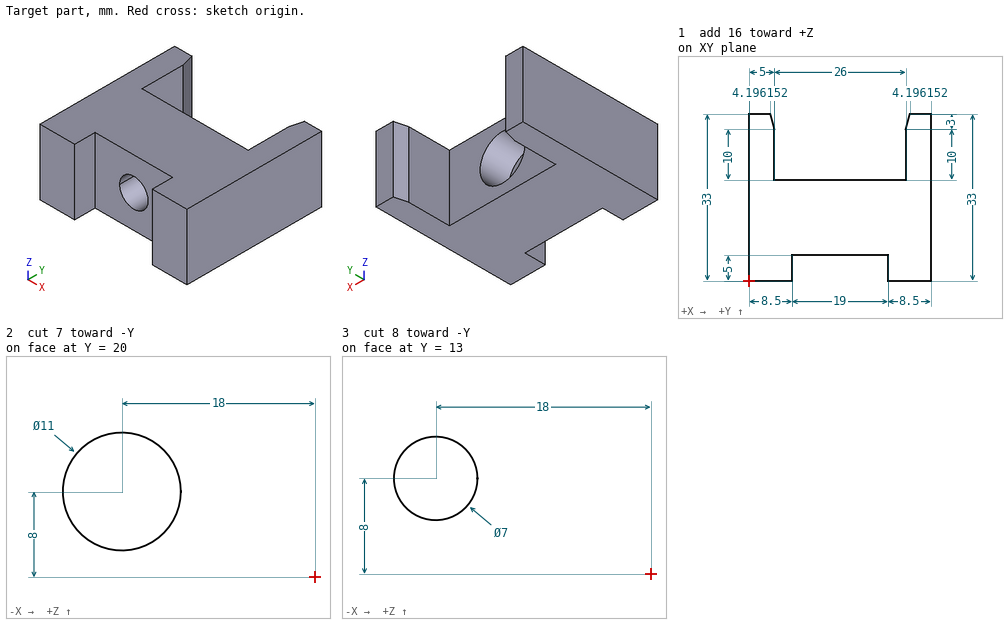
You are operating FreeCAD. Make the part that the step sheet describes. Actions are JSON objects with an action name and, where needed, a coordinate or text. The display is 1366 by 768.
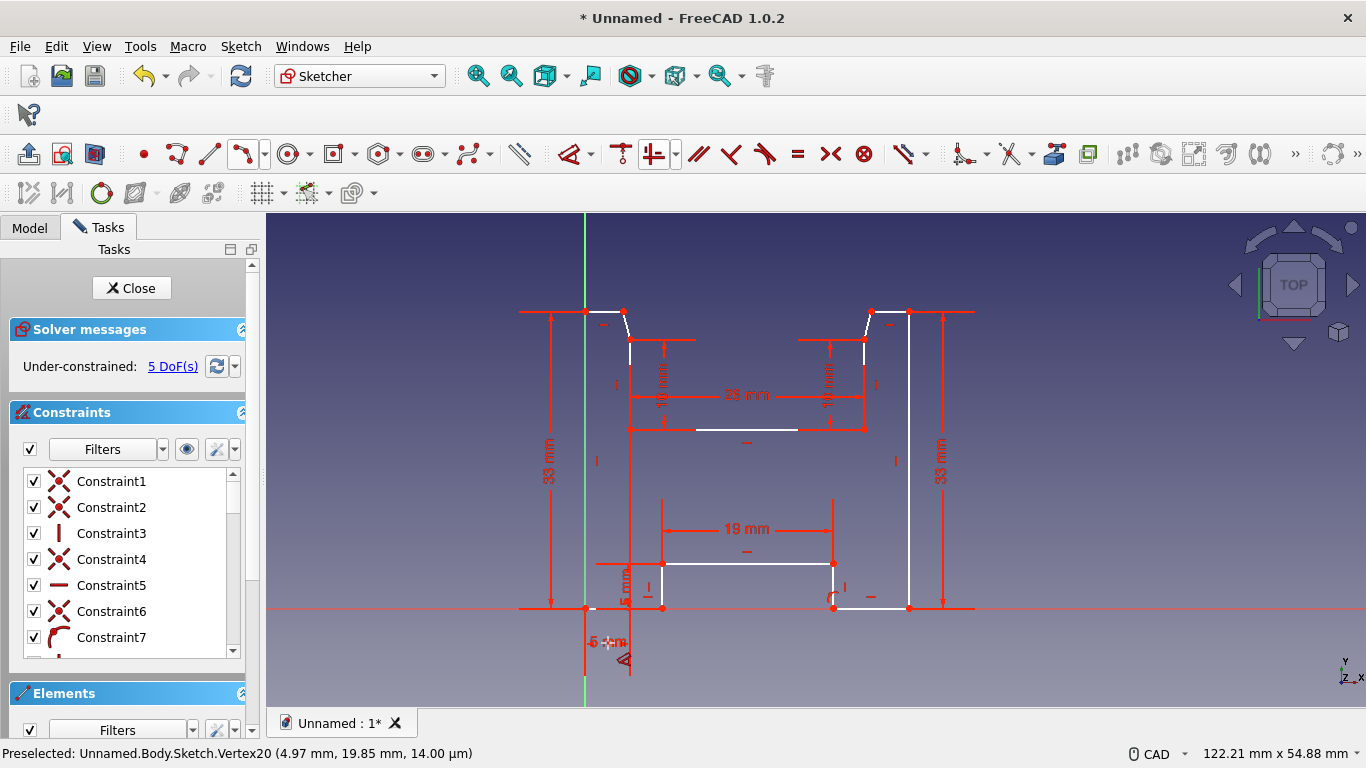
{"action": "scroll", "coordinate": [868, 323], "scroll_direction": "up", "scroll_amount": 2}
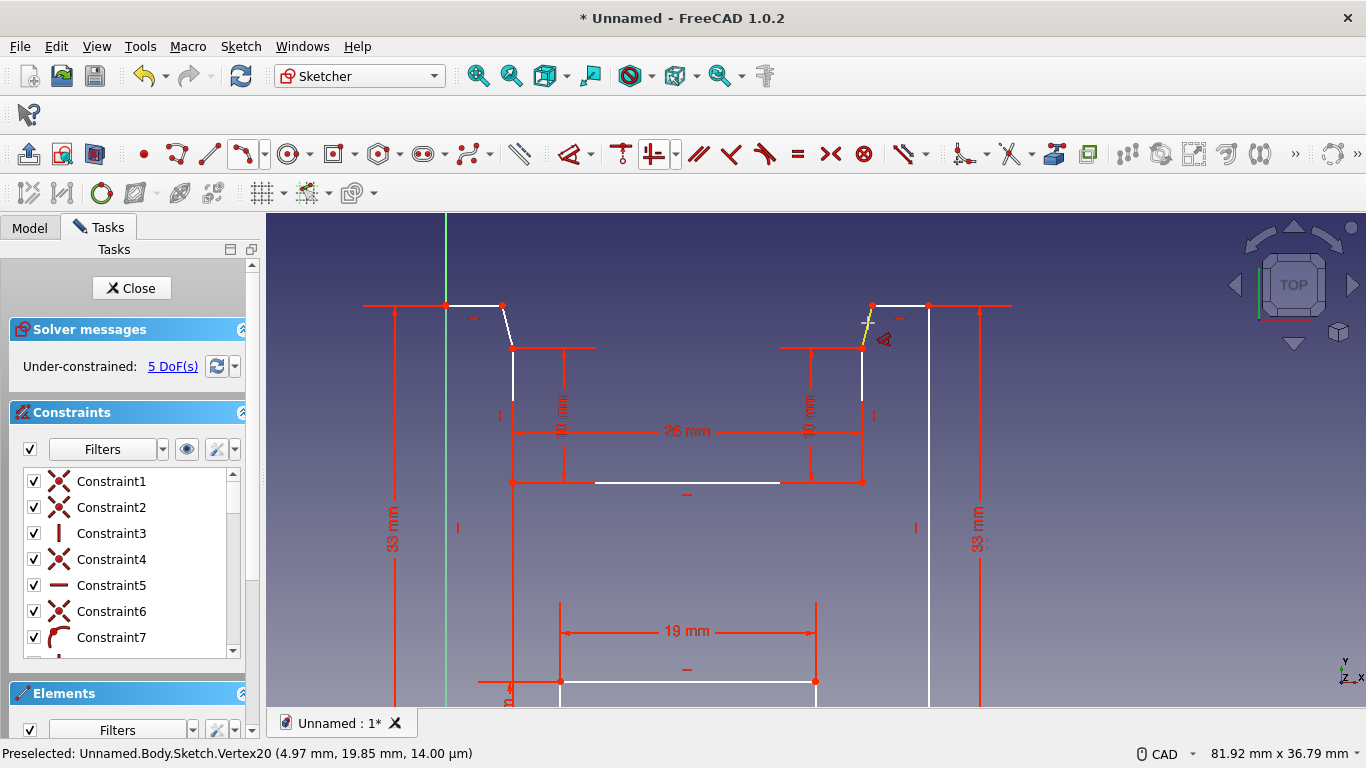
{"action": "left_click", "coordinate": [868, 323]}
{"action": "left_click", "coordinate": [906, 327]}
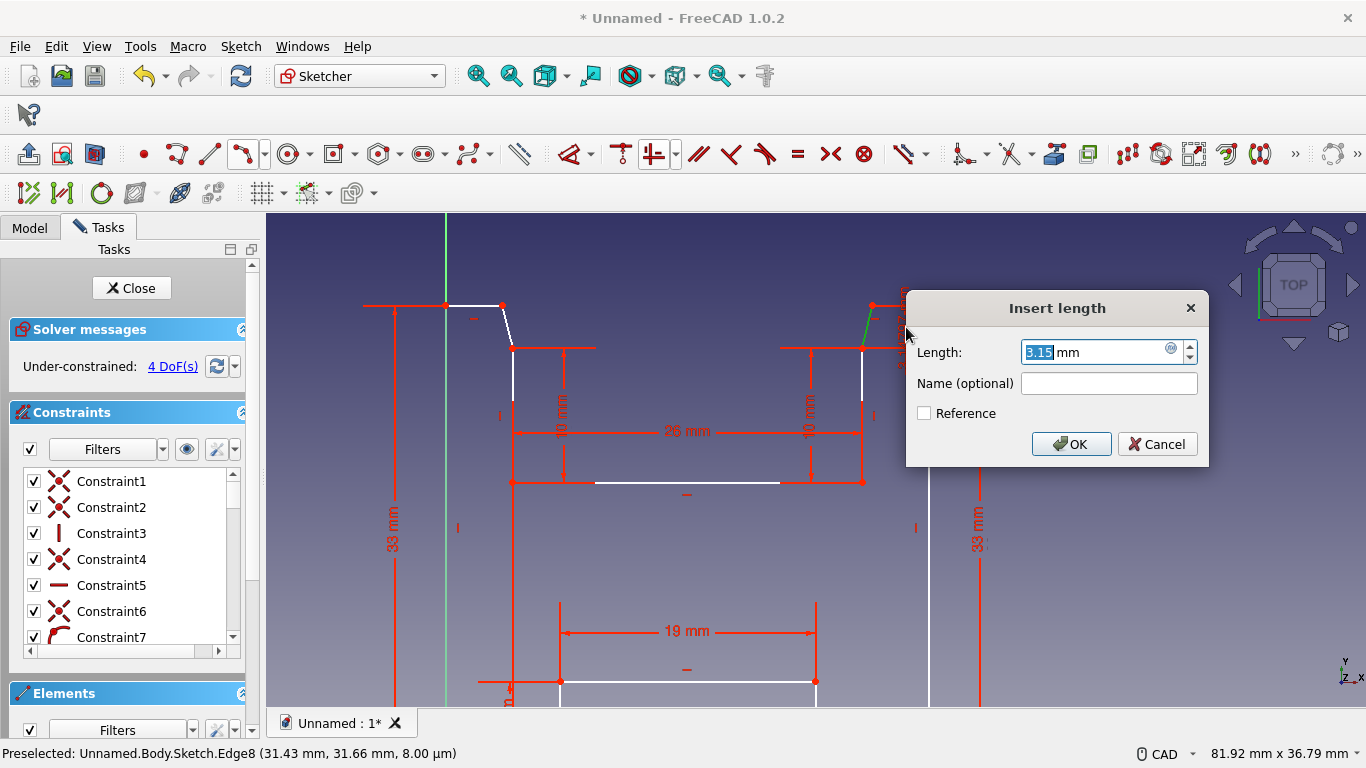
{"action": "type", "text": "3"}
{"action": "key", "text": "Return"}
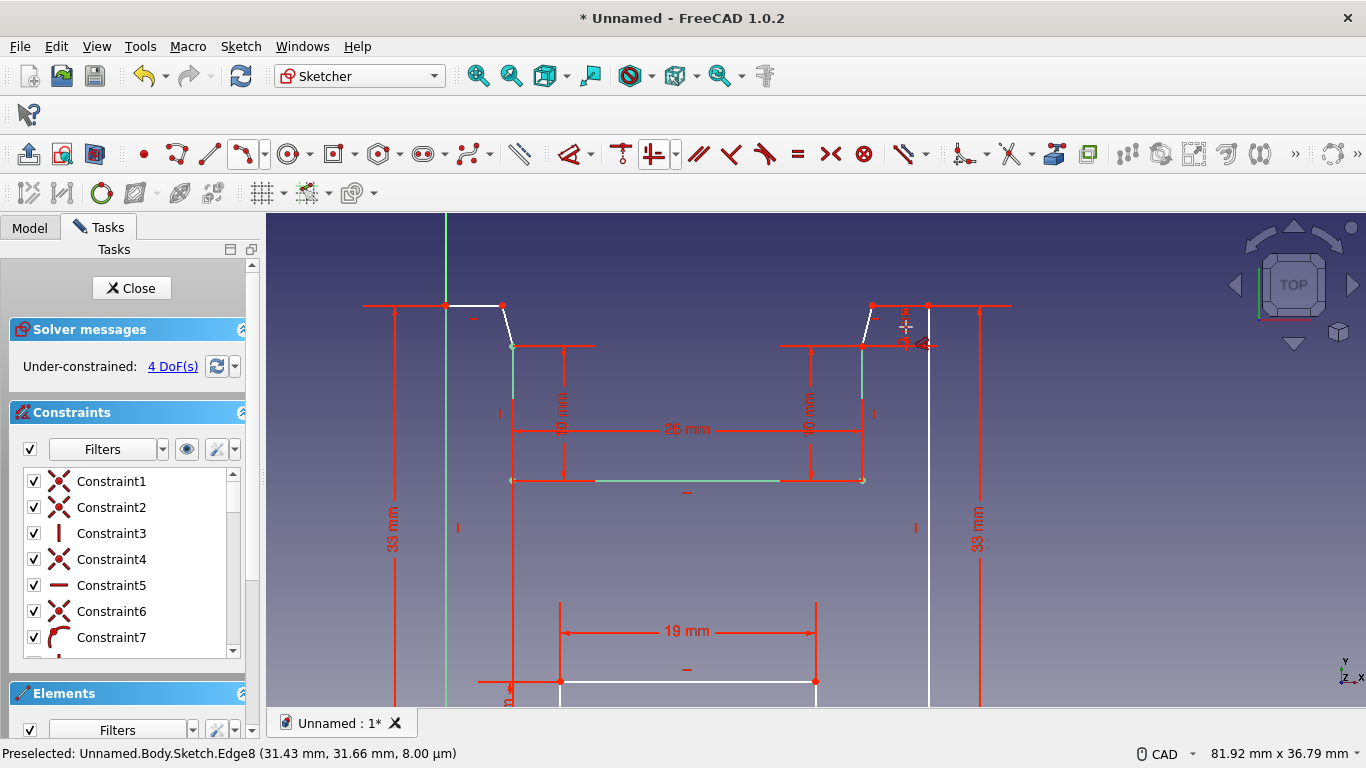
{"action": "scroll", "coordinate": [869, 323], "scroll_direction": "down", "scroll_amount": 2}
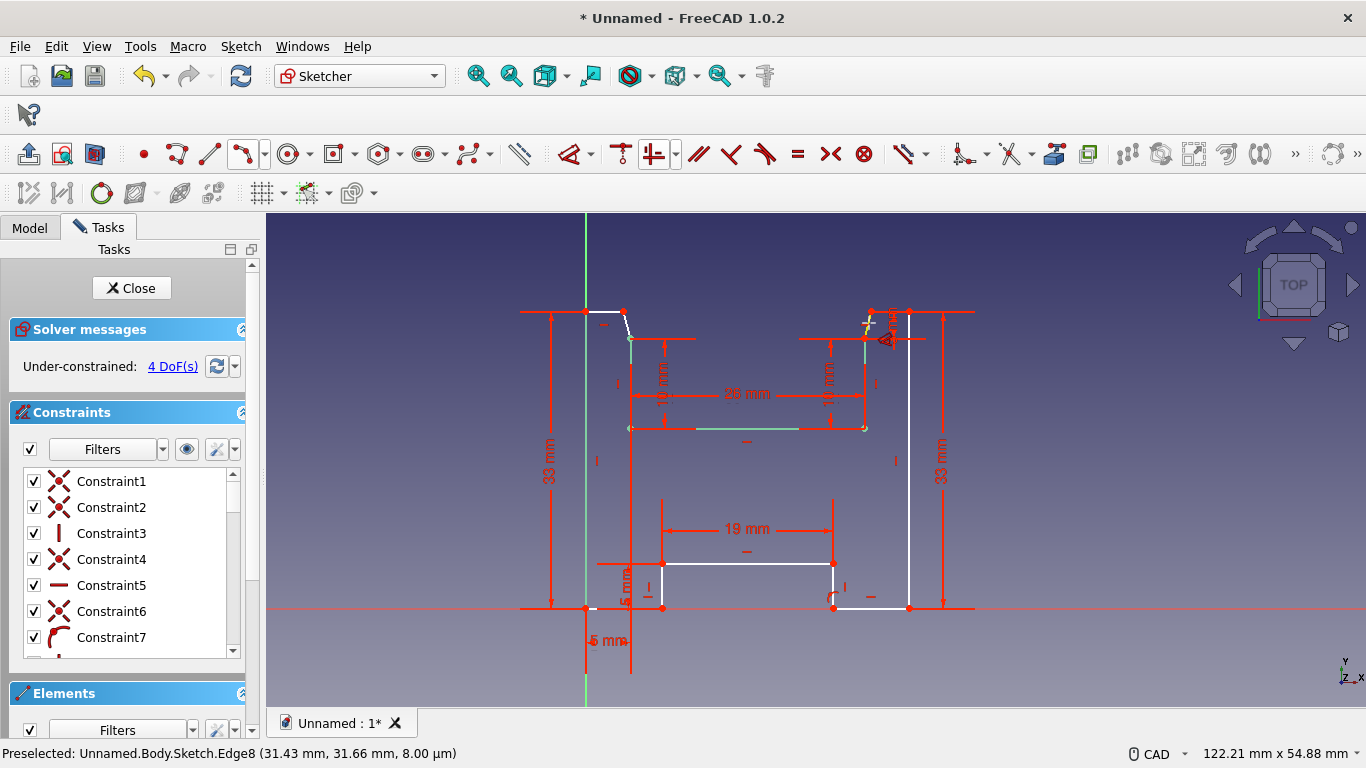
{"action": "left_click", "coordinate": [609, 609]}
{"action": "left_click", "coordinate": [624, 667]}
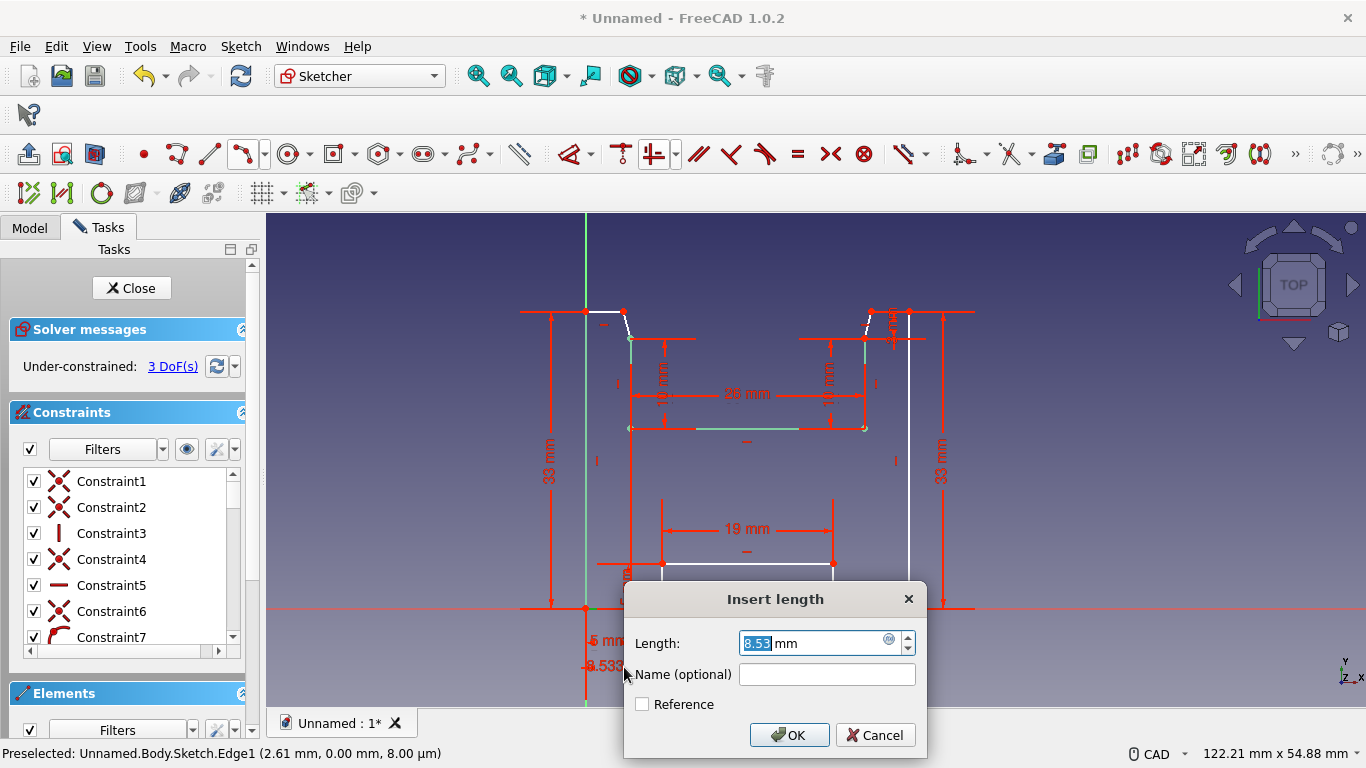
{"action": "type", "text": "8.5"}
{"action": "key", "text": "Return"}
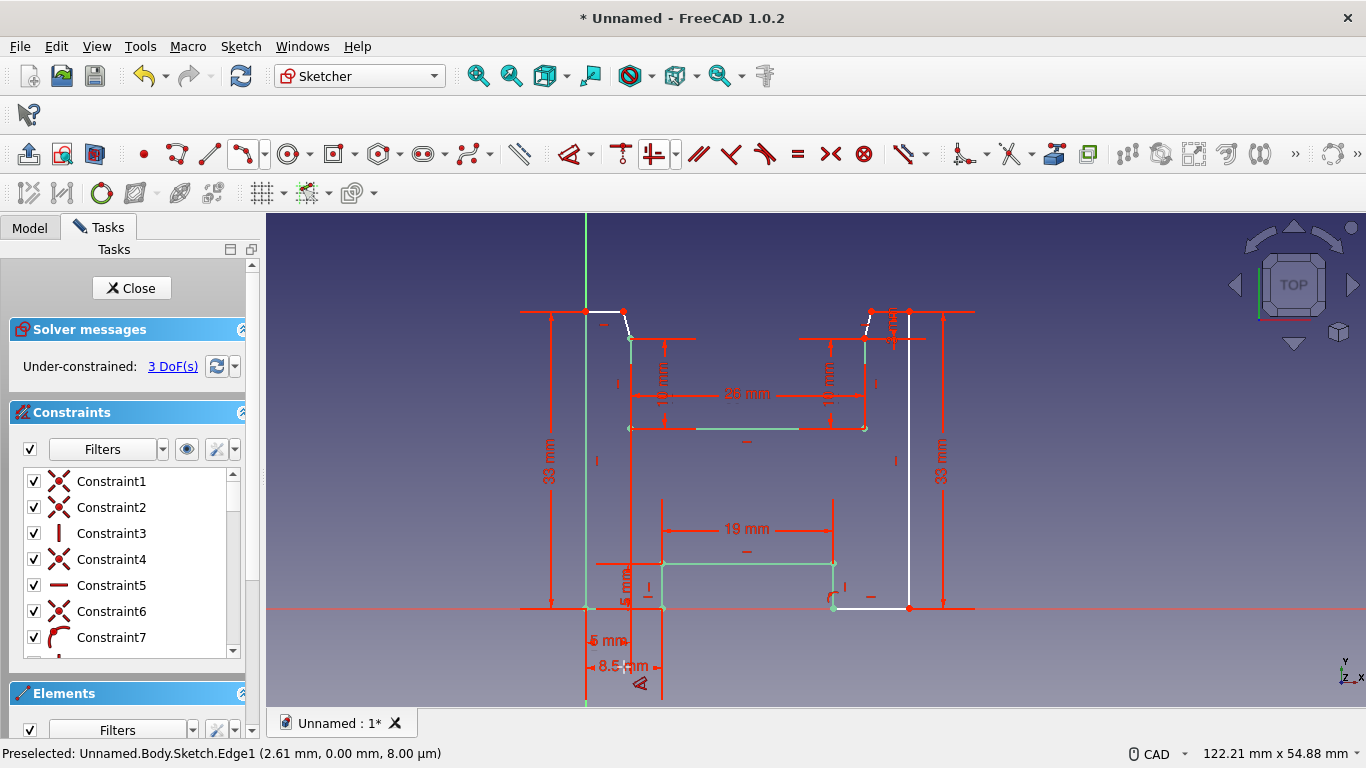
{"action": "left_click", "coordinate": [856, 609]}
{"action": "left_click", "coordinate": [871, 643]}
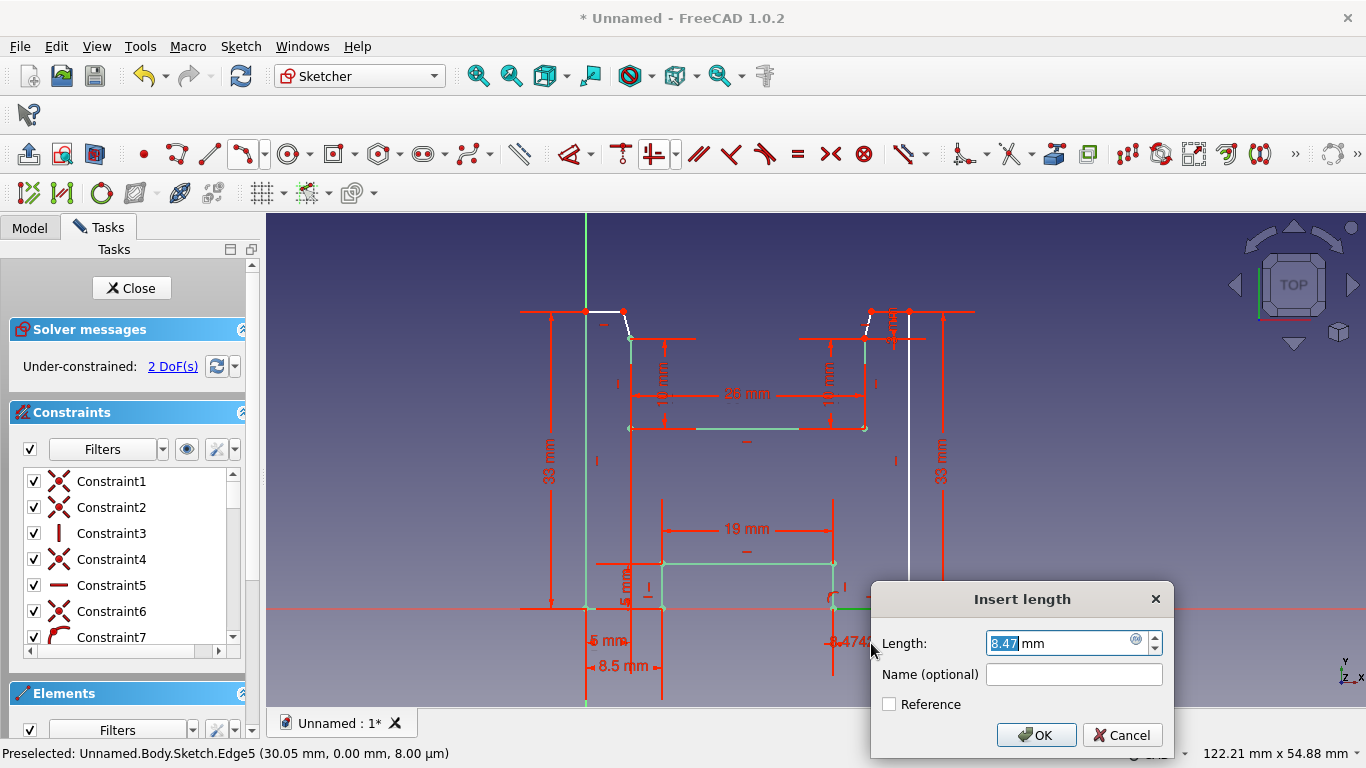
{"action": "type", "text": "8.5"}
{"action": "key", "text": "Return"}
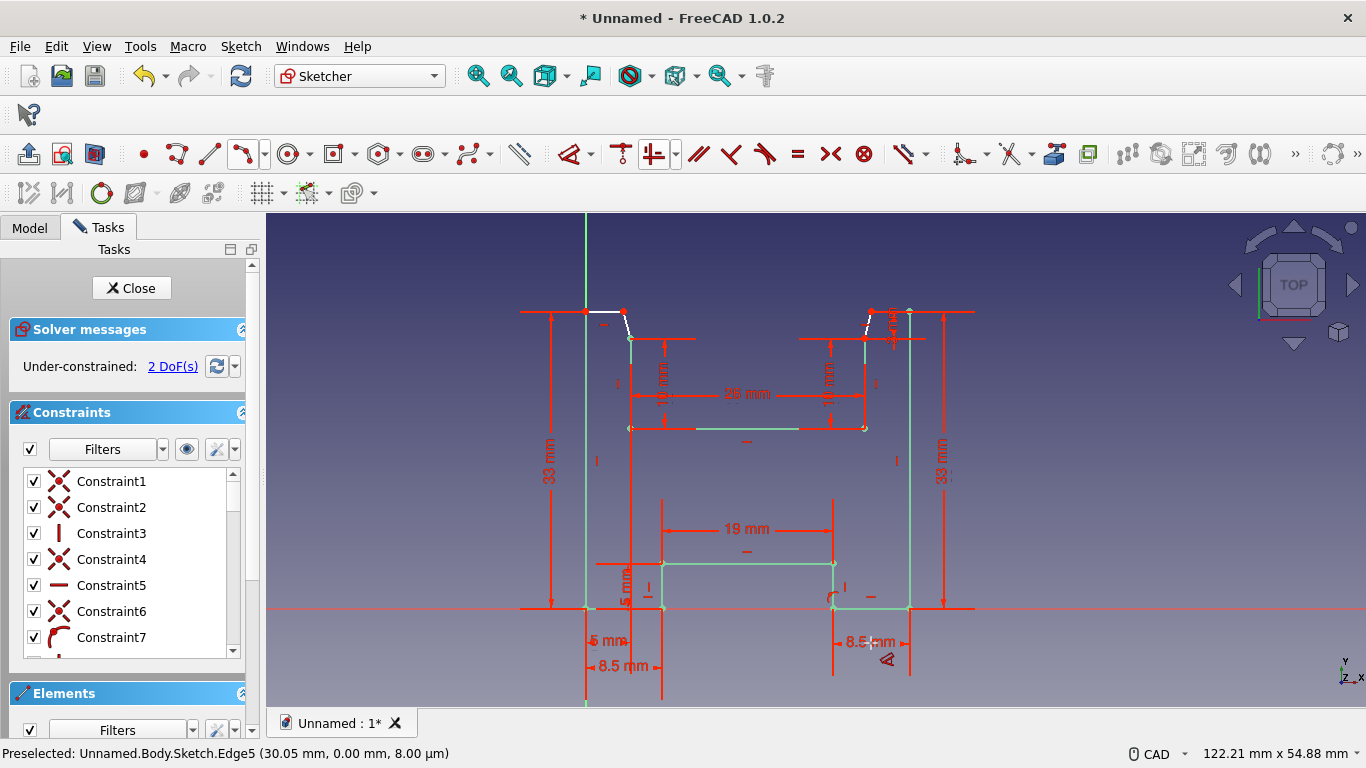
{"action": "left_click", "coordinate": [898, 312]}
{"action": "left_click", "coordinate": [890, 278]}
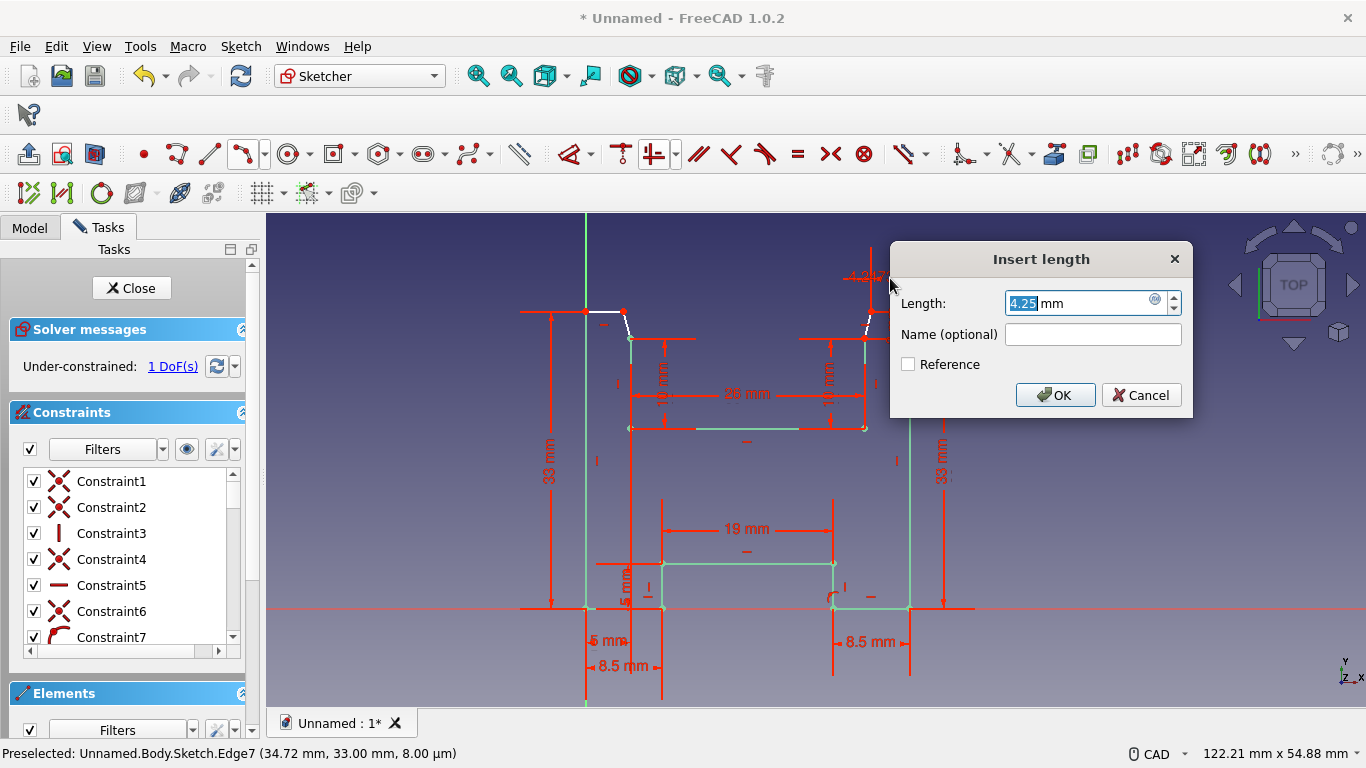
{"action": "type", "text": "4.196152"}
{"action": "key", "text": "Return"}